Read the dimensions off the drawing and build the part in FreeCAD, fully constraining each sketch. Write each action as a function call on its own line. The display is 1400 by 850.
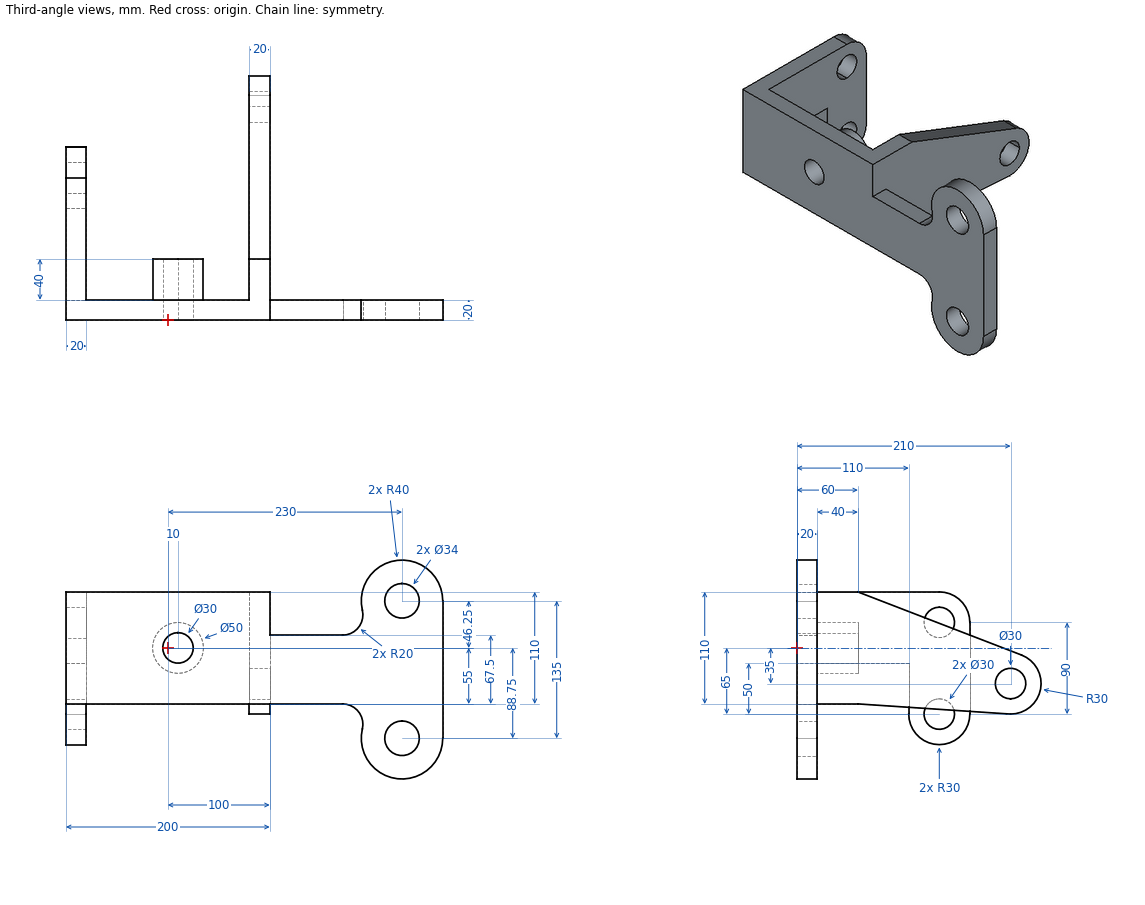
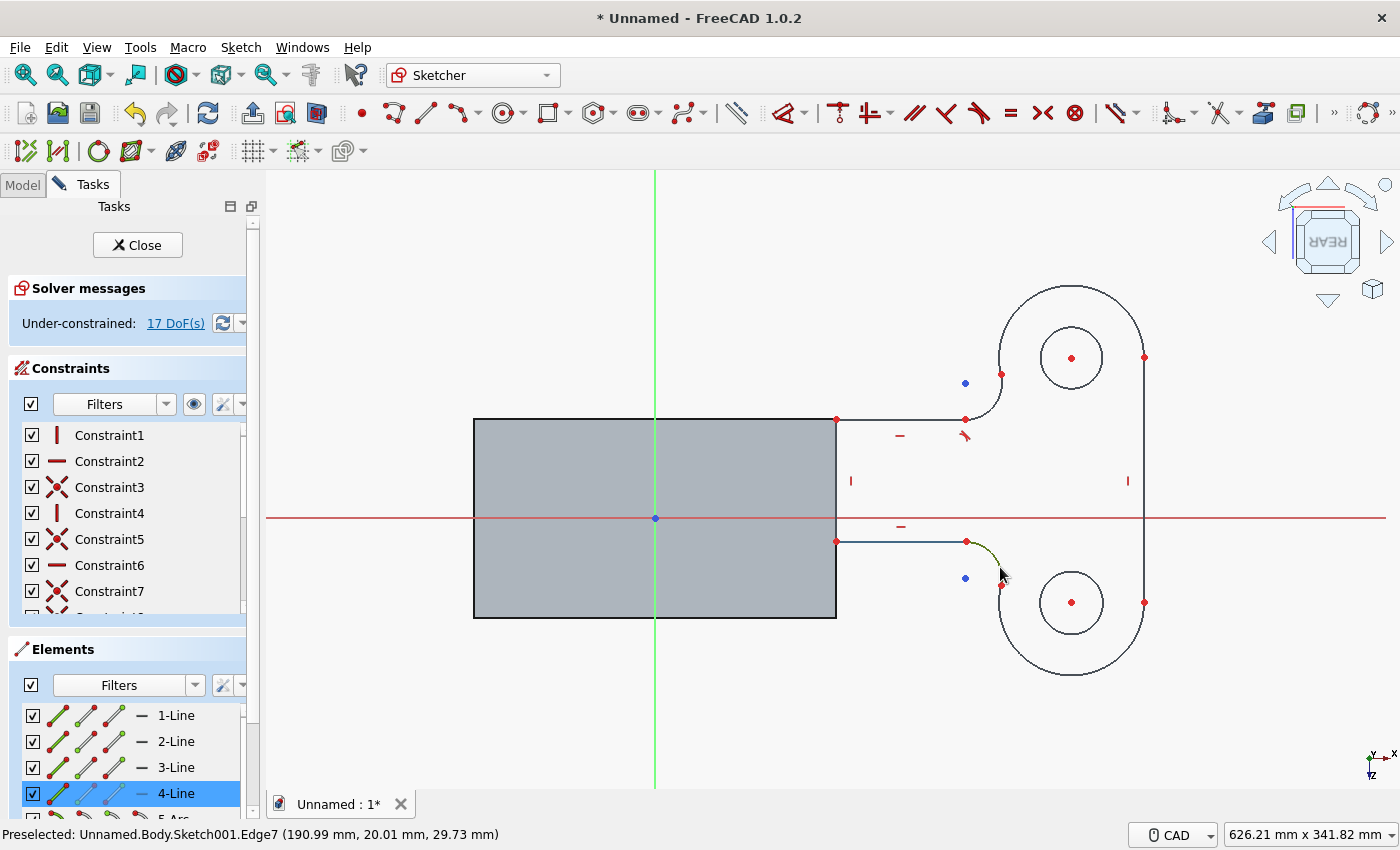
key(t)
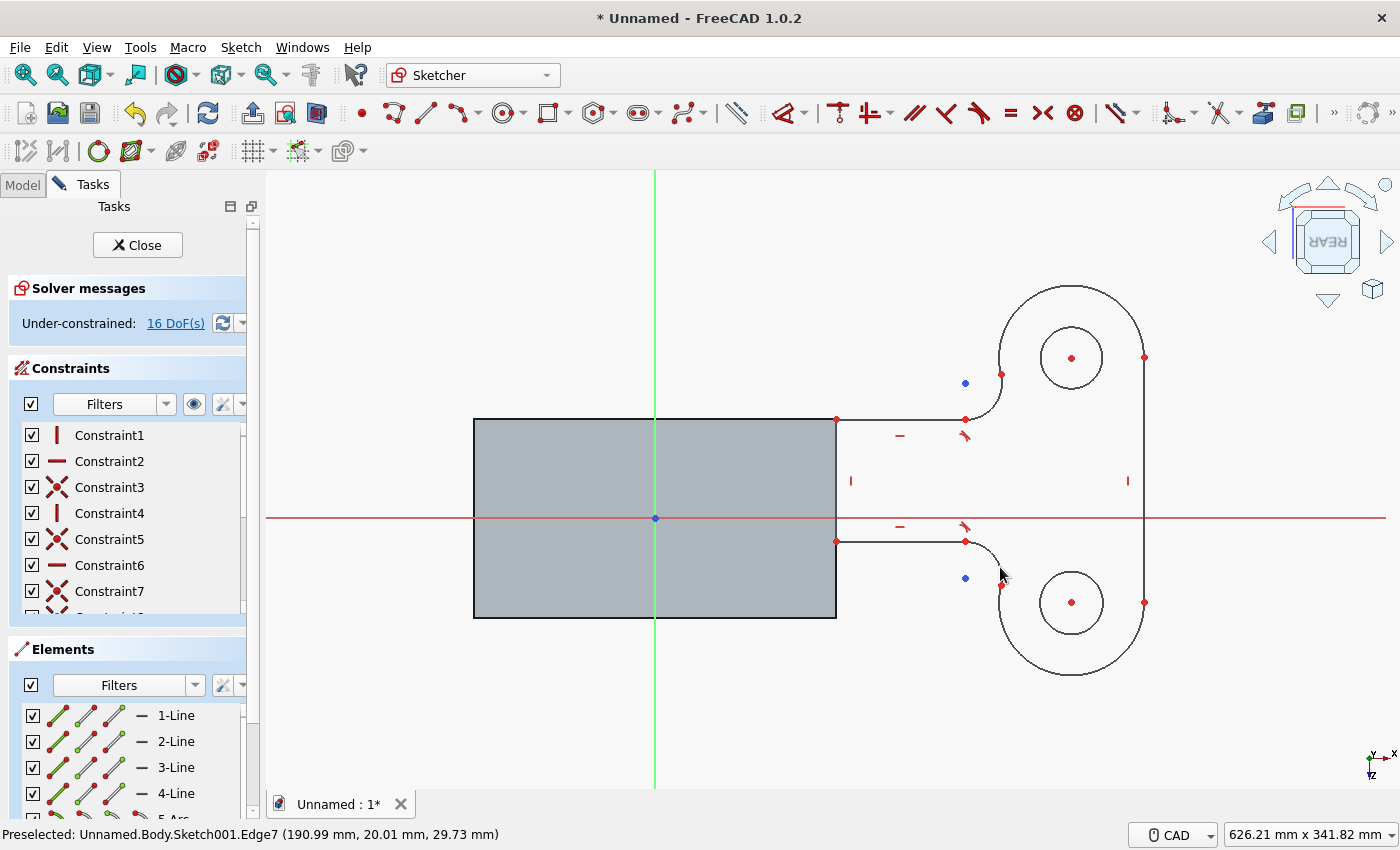
click(1110, 296)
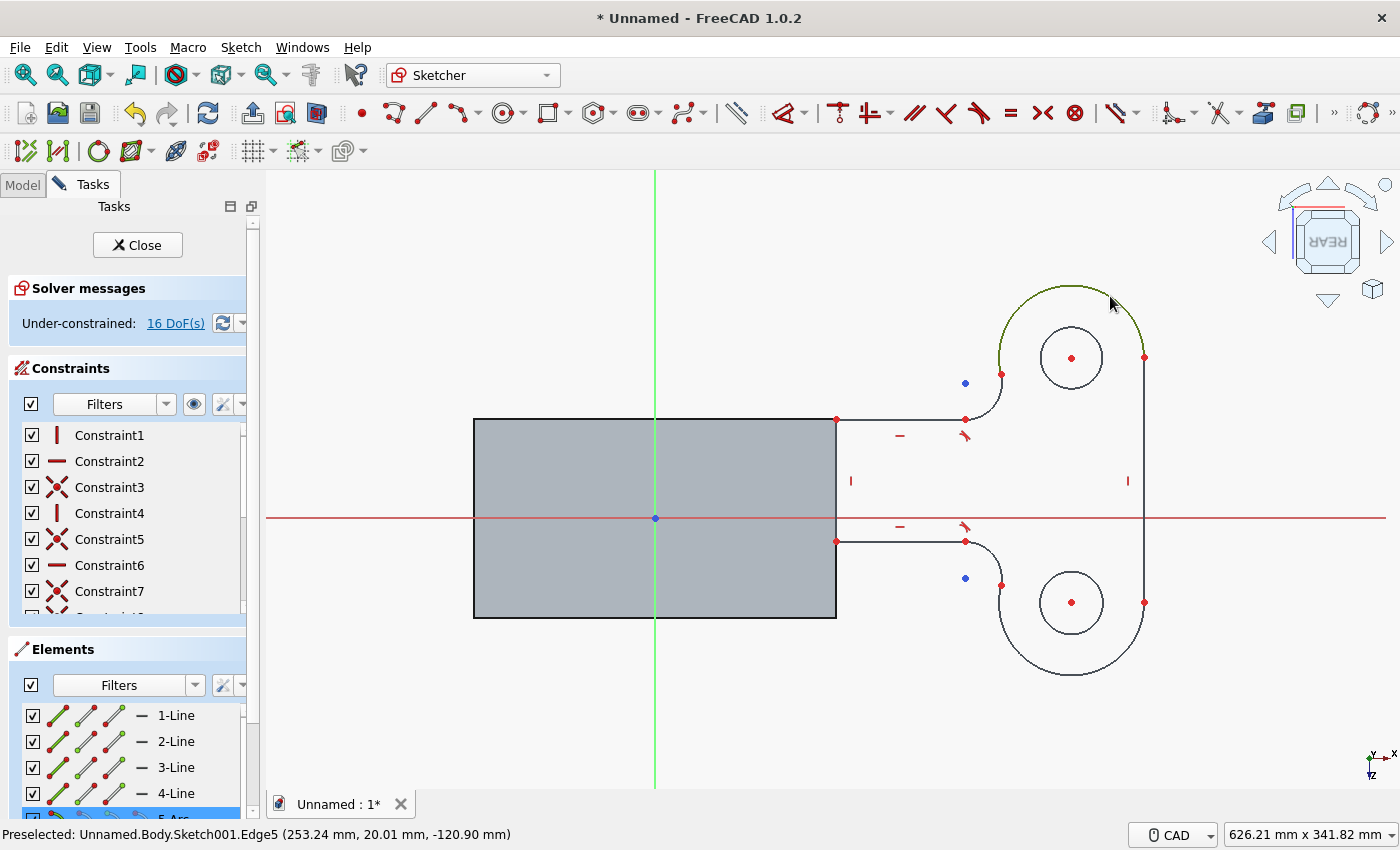
click(984, 415)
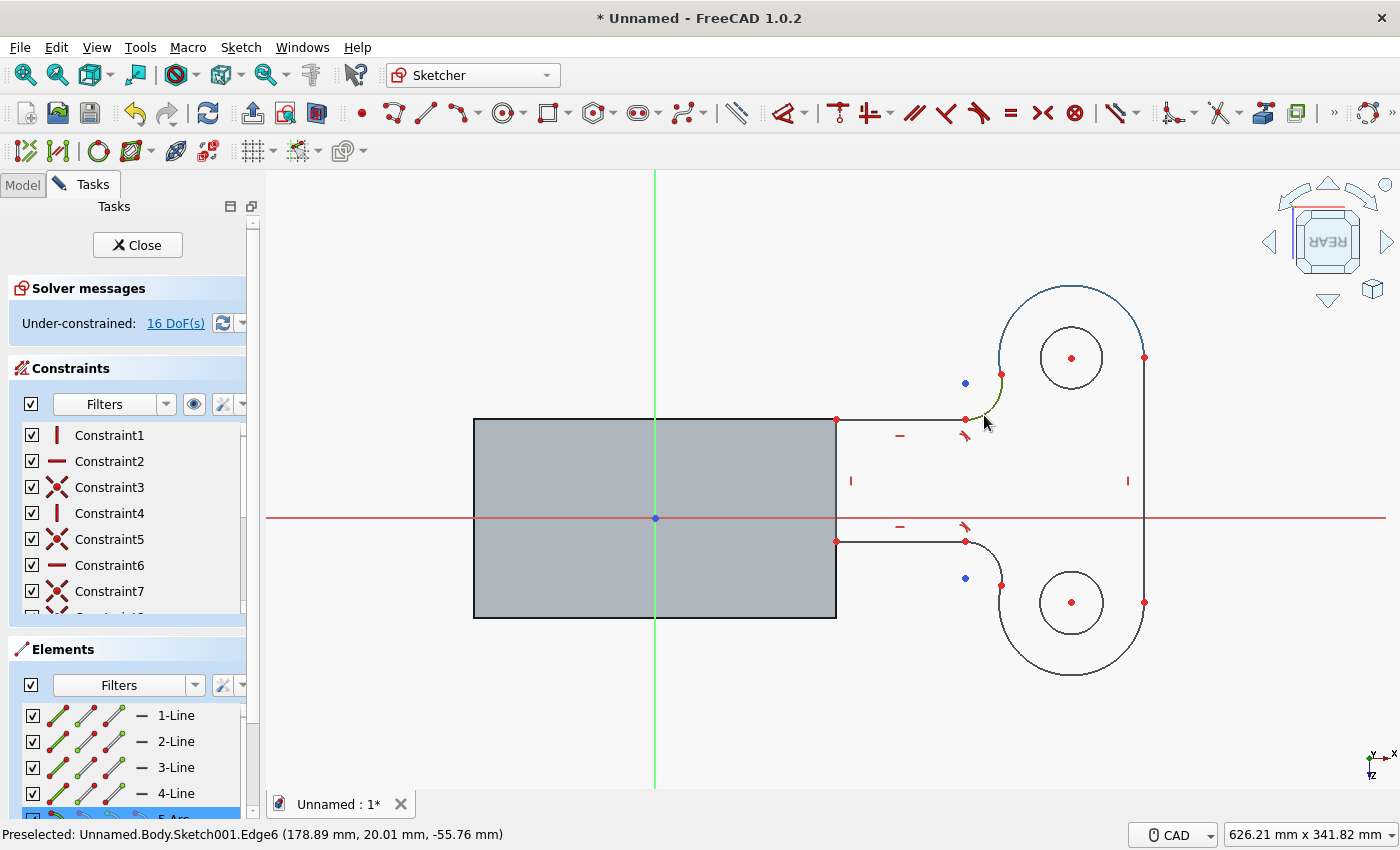
click(980, 114)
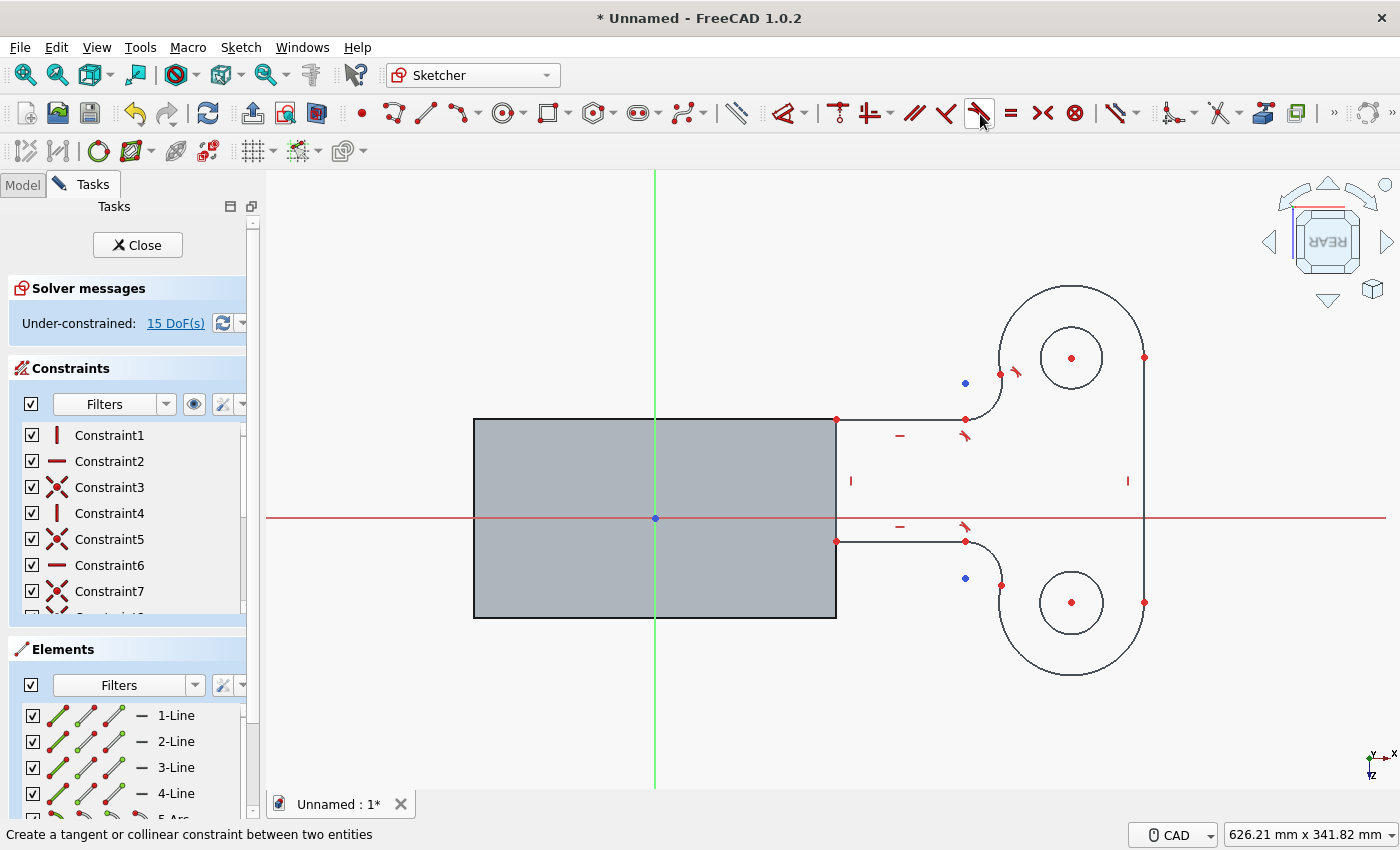
click(1000, 567)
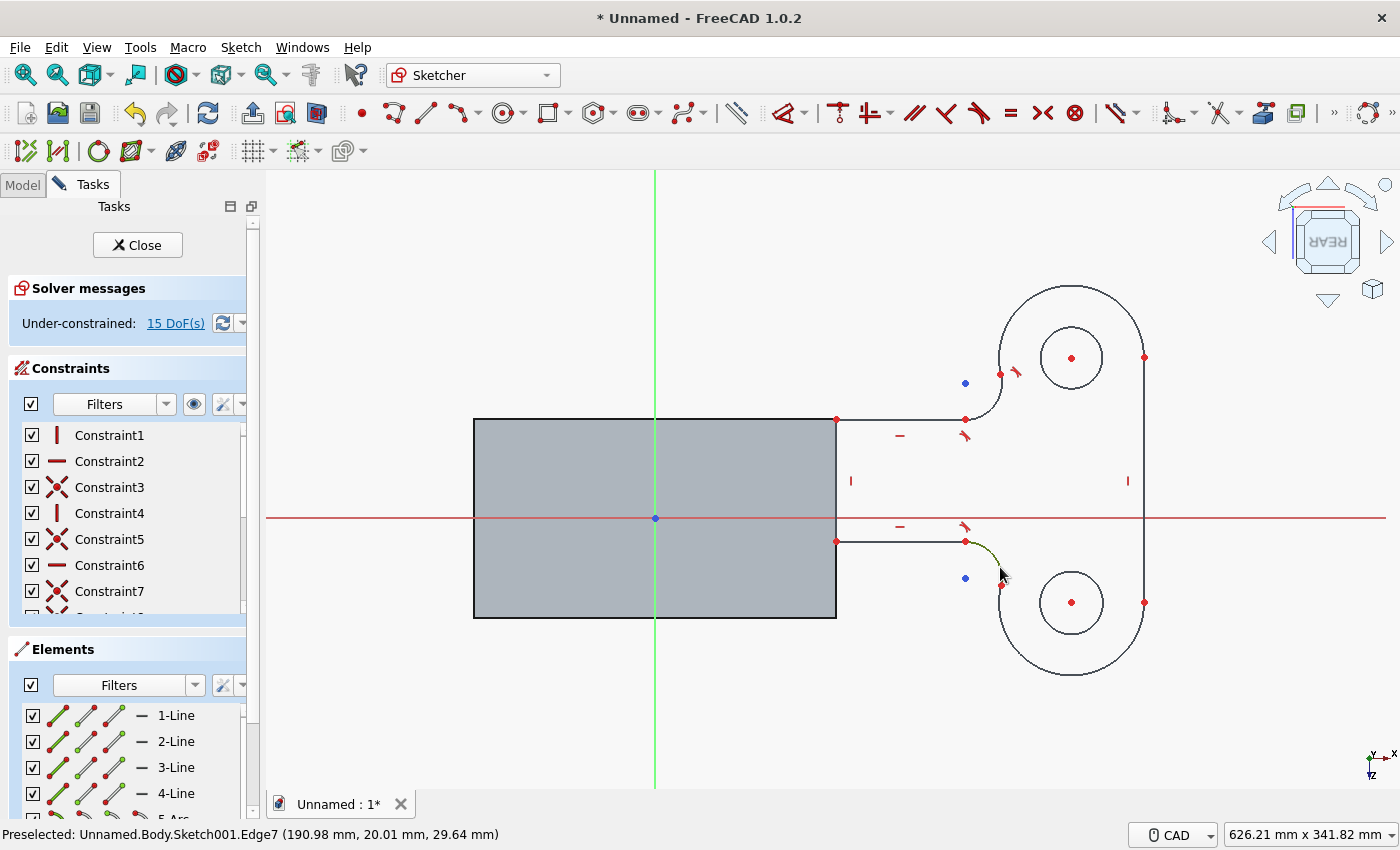
click(1020, 654)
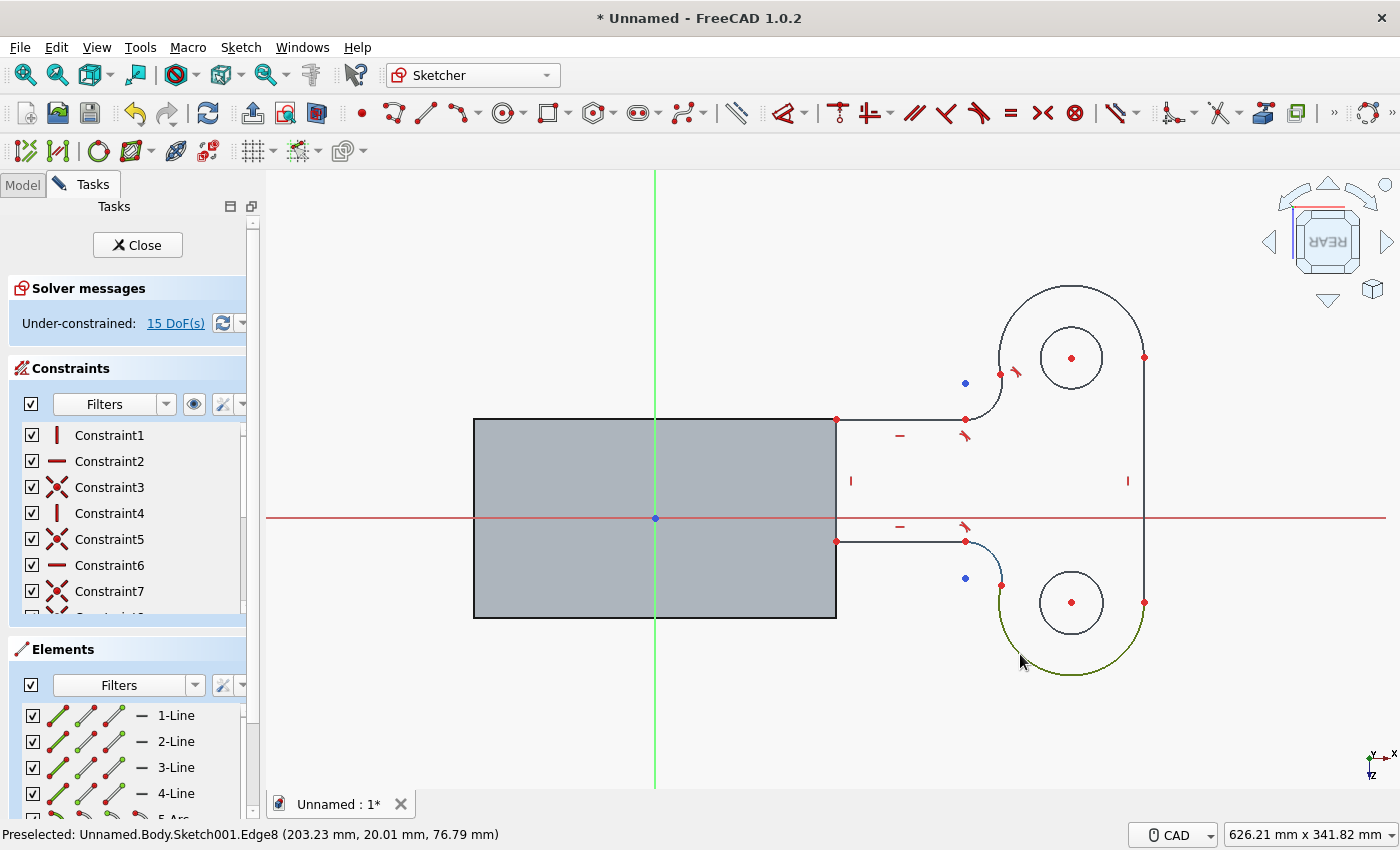
click(980, 114)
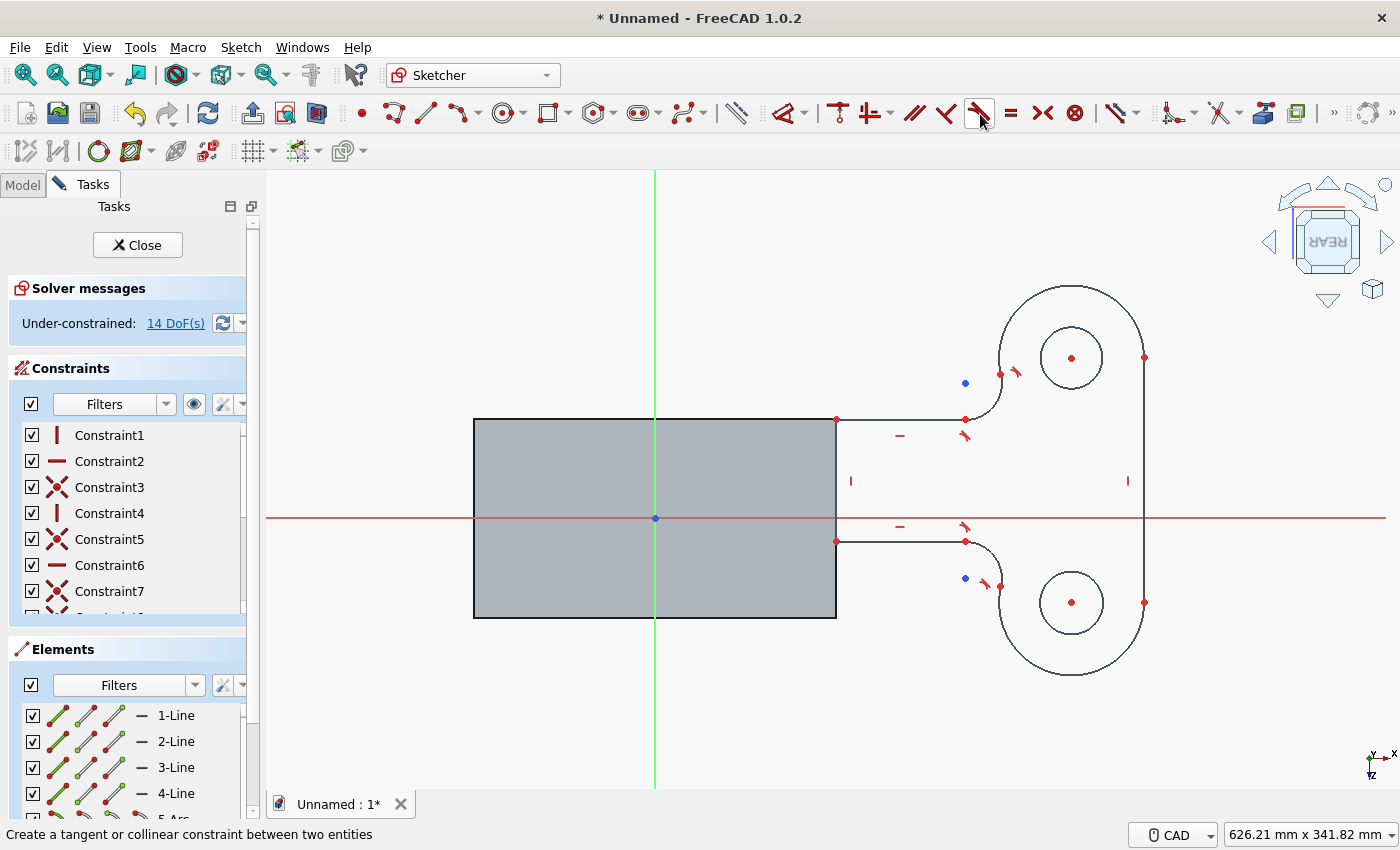
click(984, 415)